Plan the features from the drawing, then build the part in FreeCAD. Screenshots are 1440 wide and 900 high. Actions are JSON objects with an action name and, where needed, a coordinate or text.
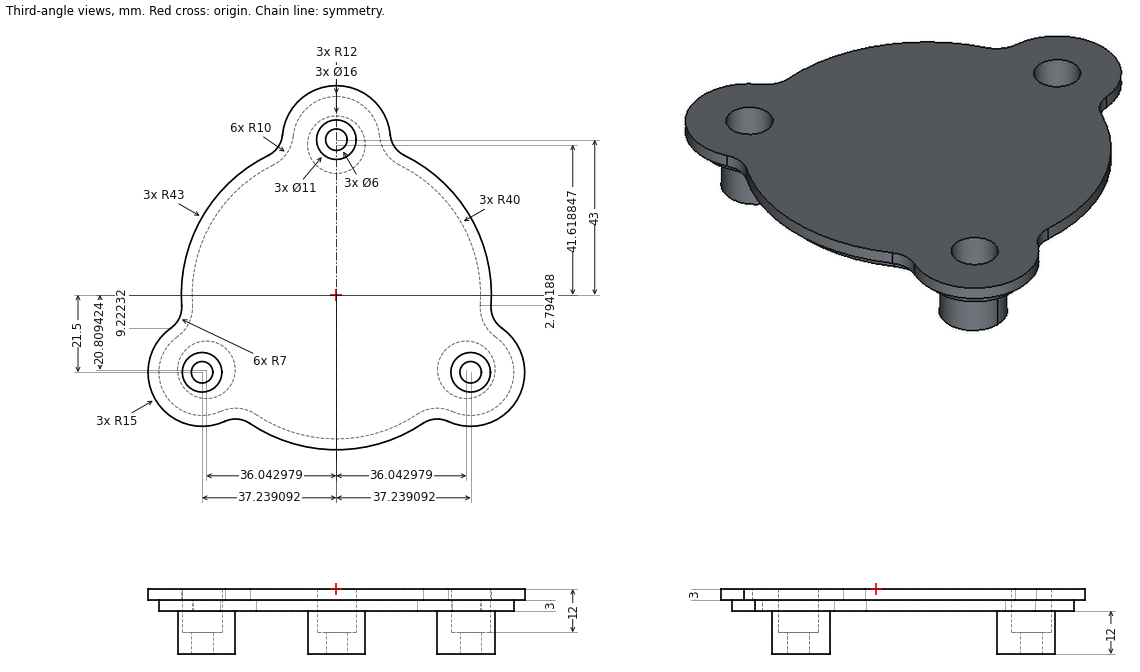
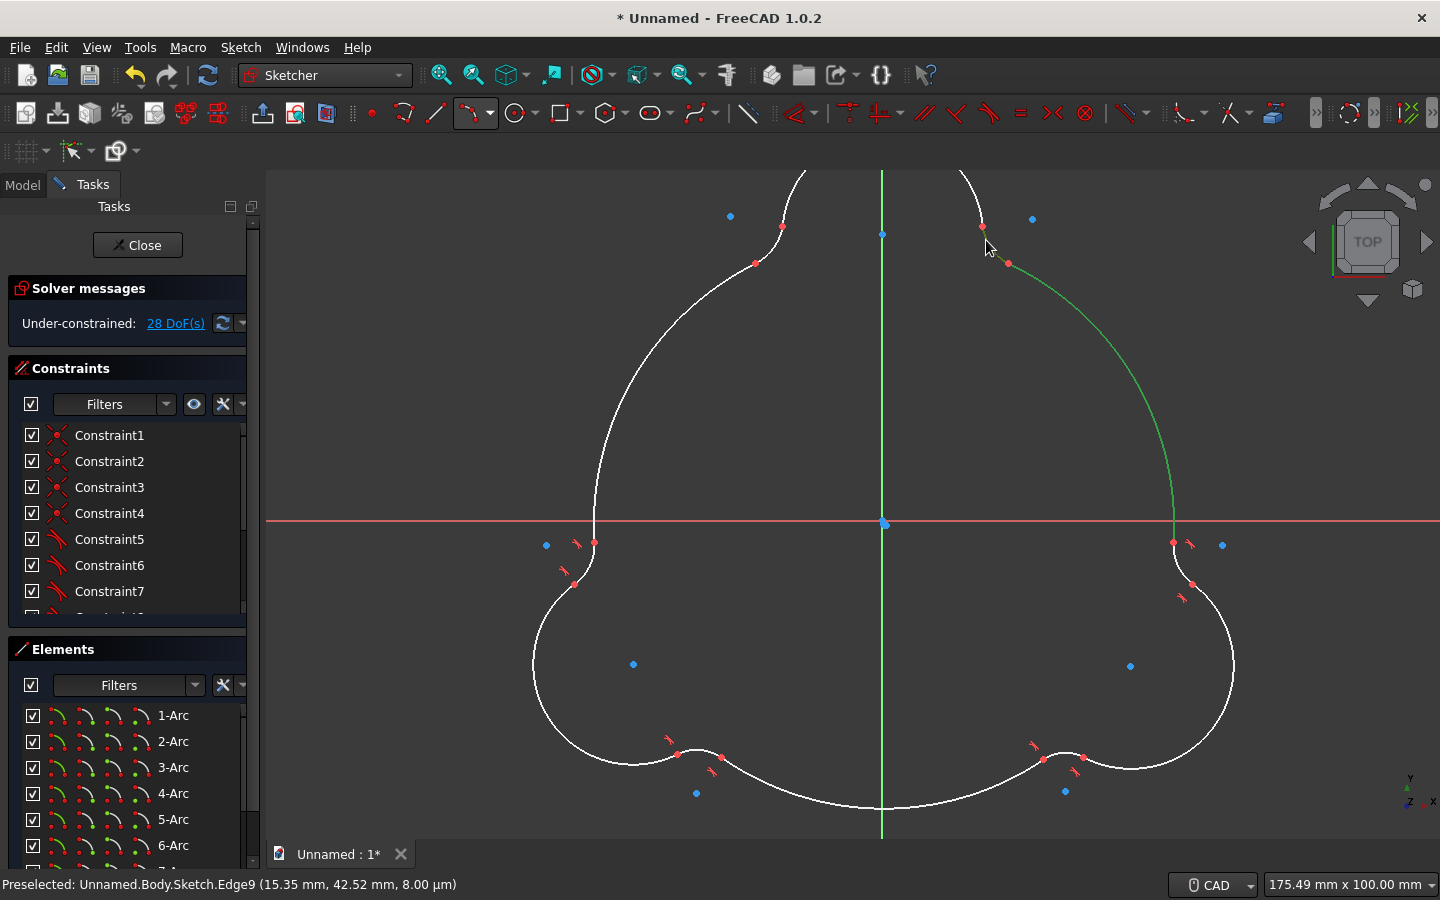
{"action": "left_click", "coordinate": [990, 114]}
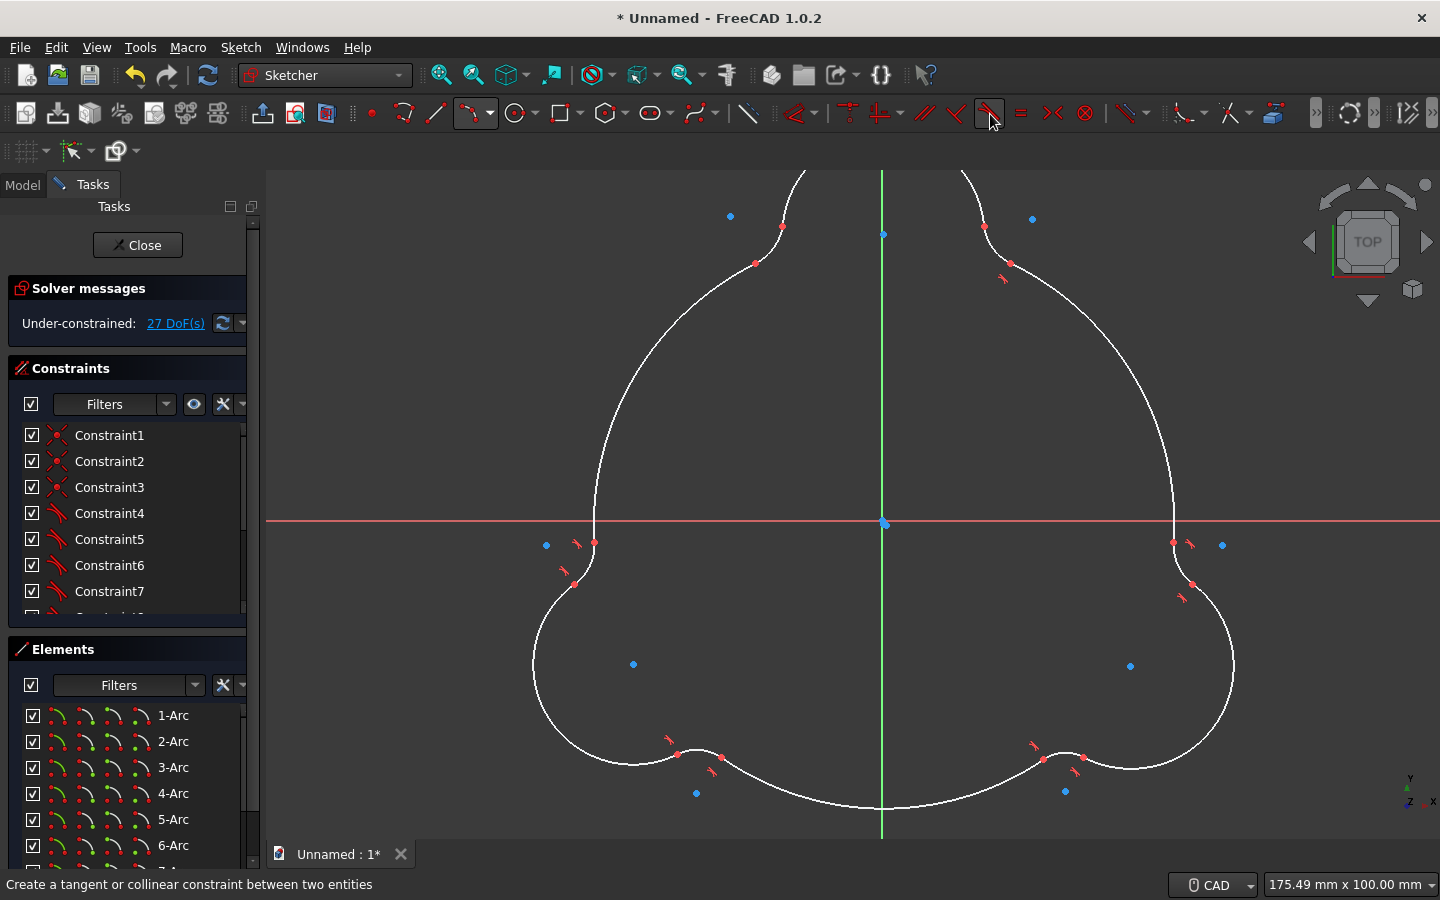
{"action": "left_click", "coordinate": [988, 240]}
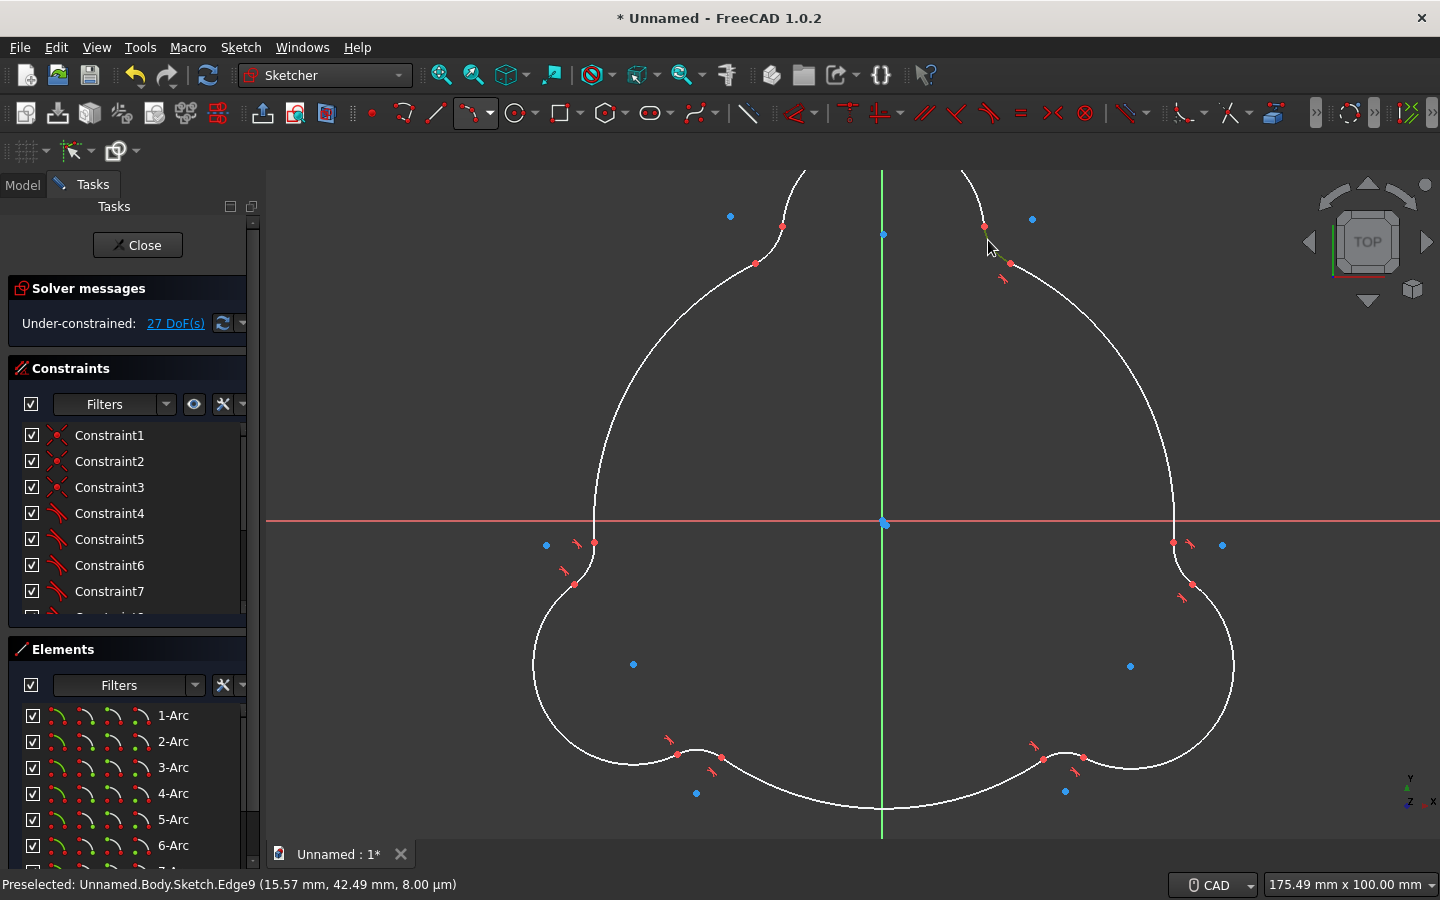
{"action": "scroll", "coordinate": [586, 574], "scroll_direction": "down", "scroll_amount": 2}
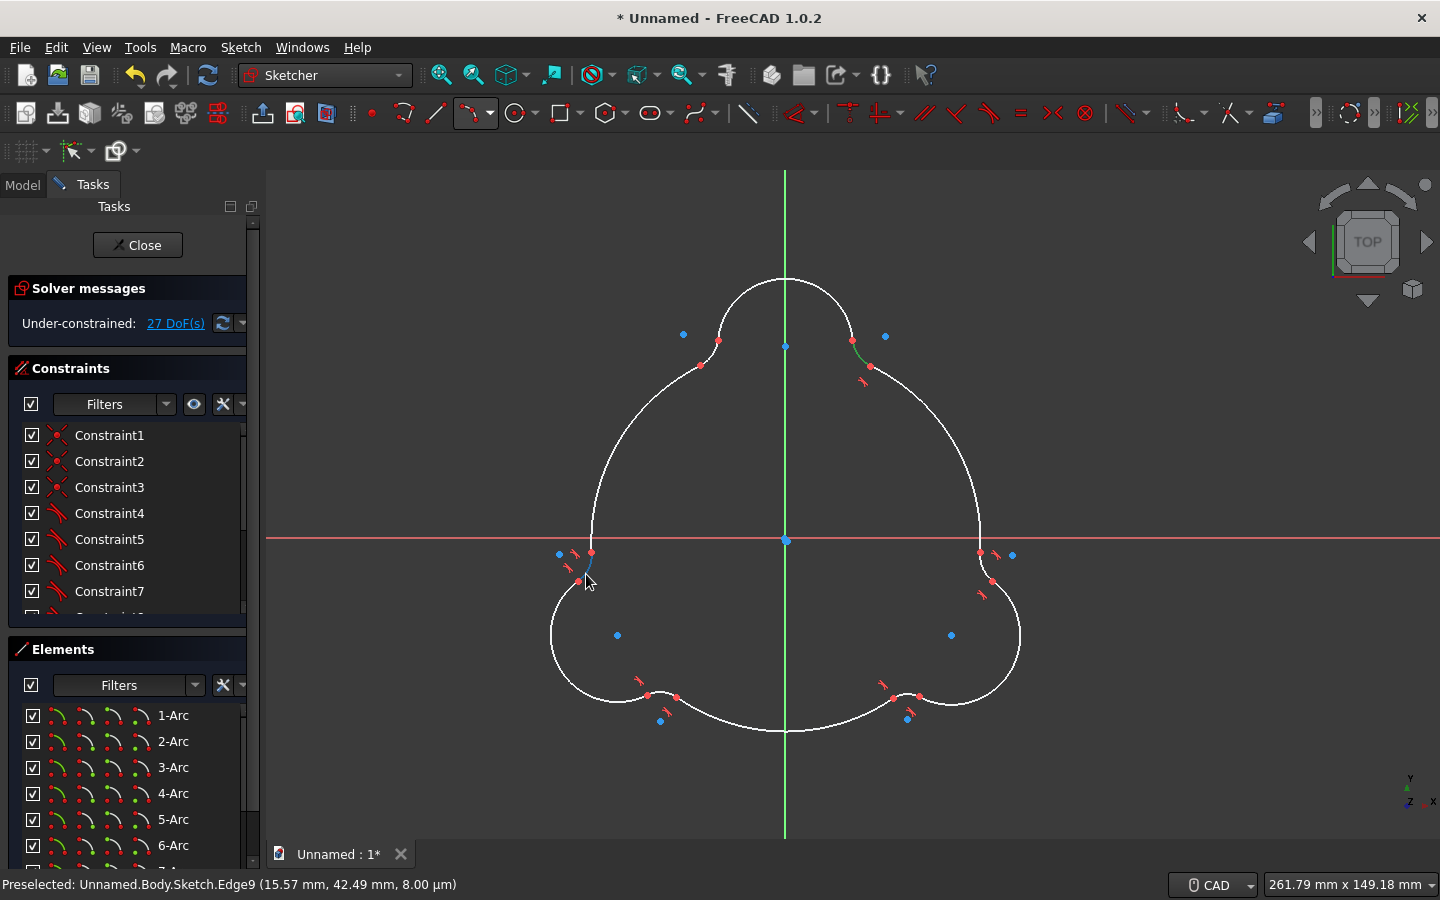
{"action": "left_click", "coordinate": [823, 290]}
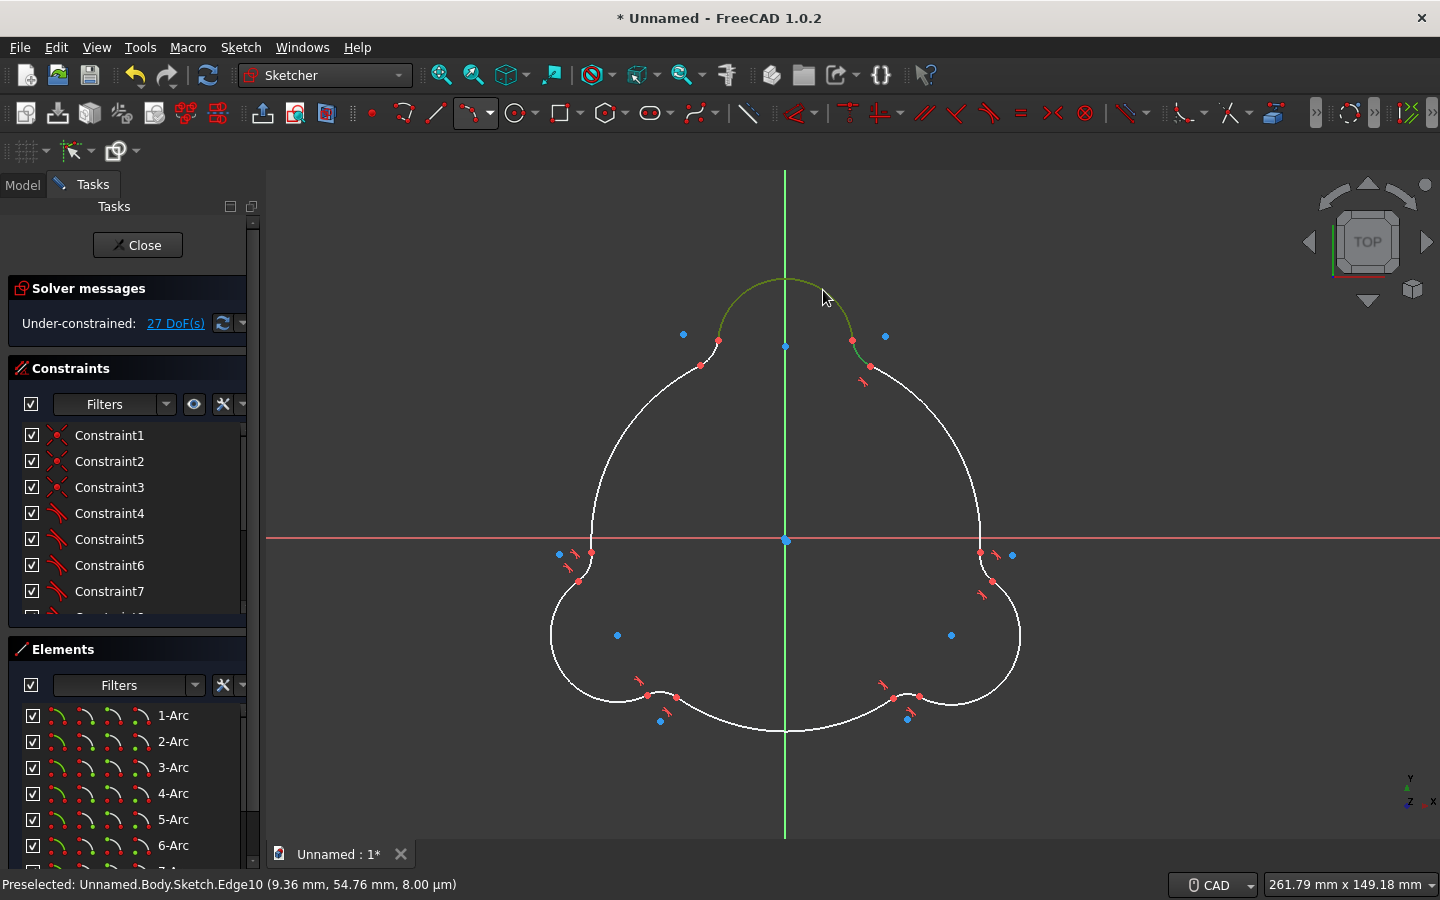
{"action": "left_click", "coordinate": [990, 114]}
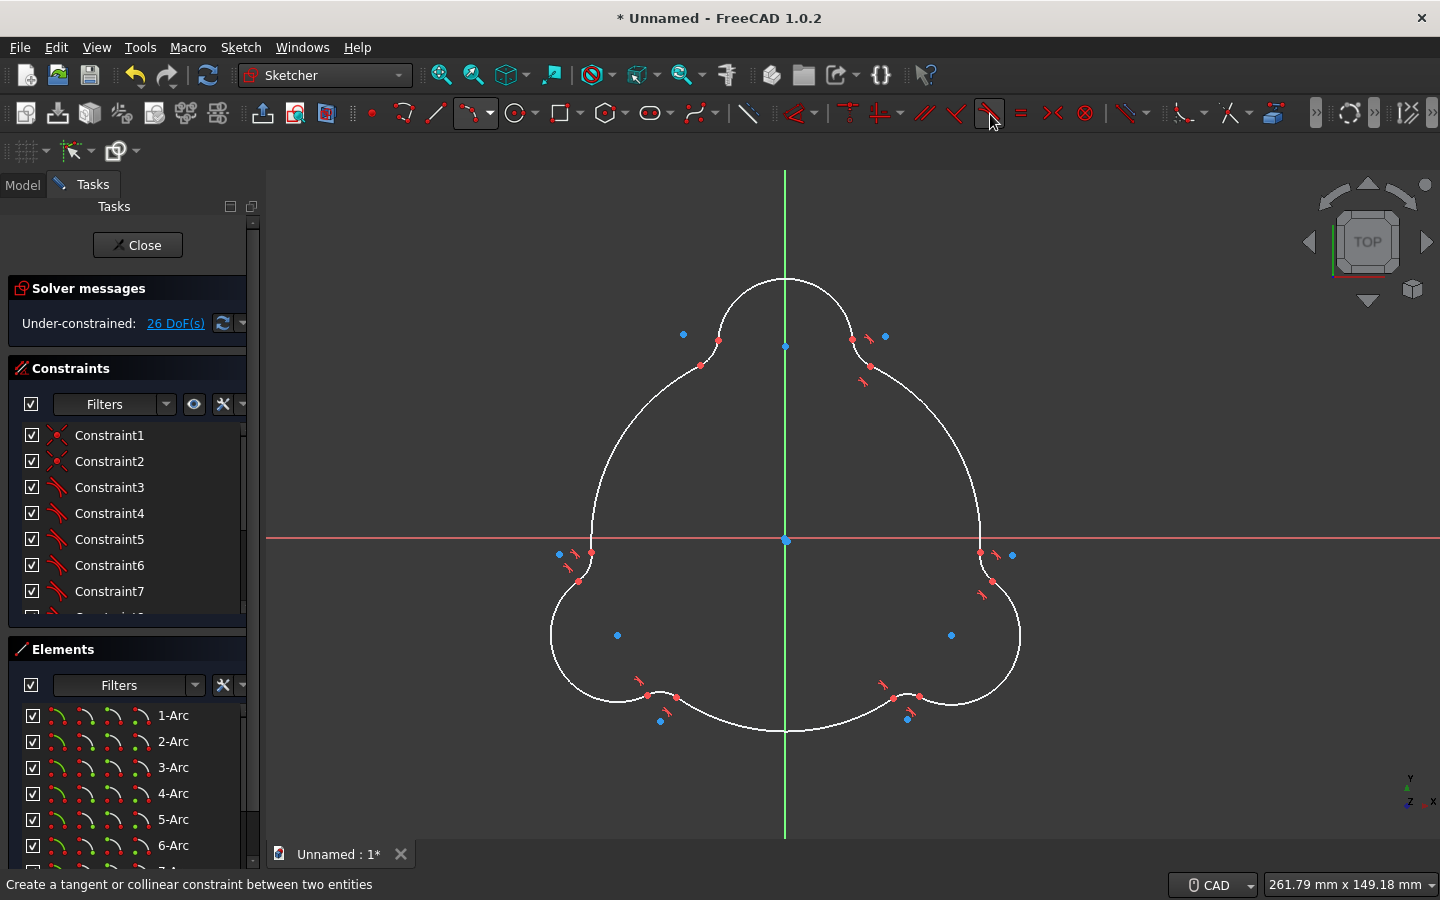
{"action": "left_click", "coordinate": [823, 290]}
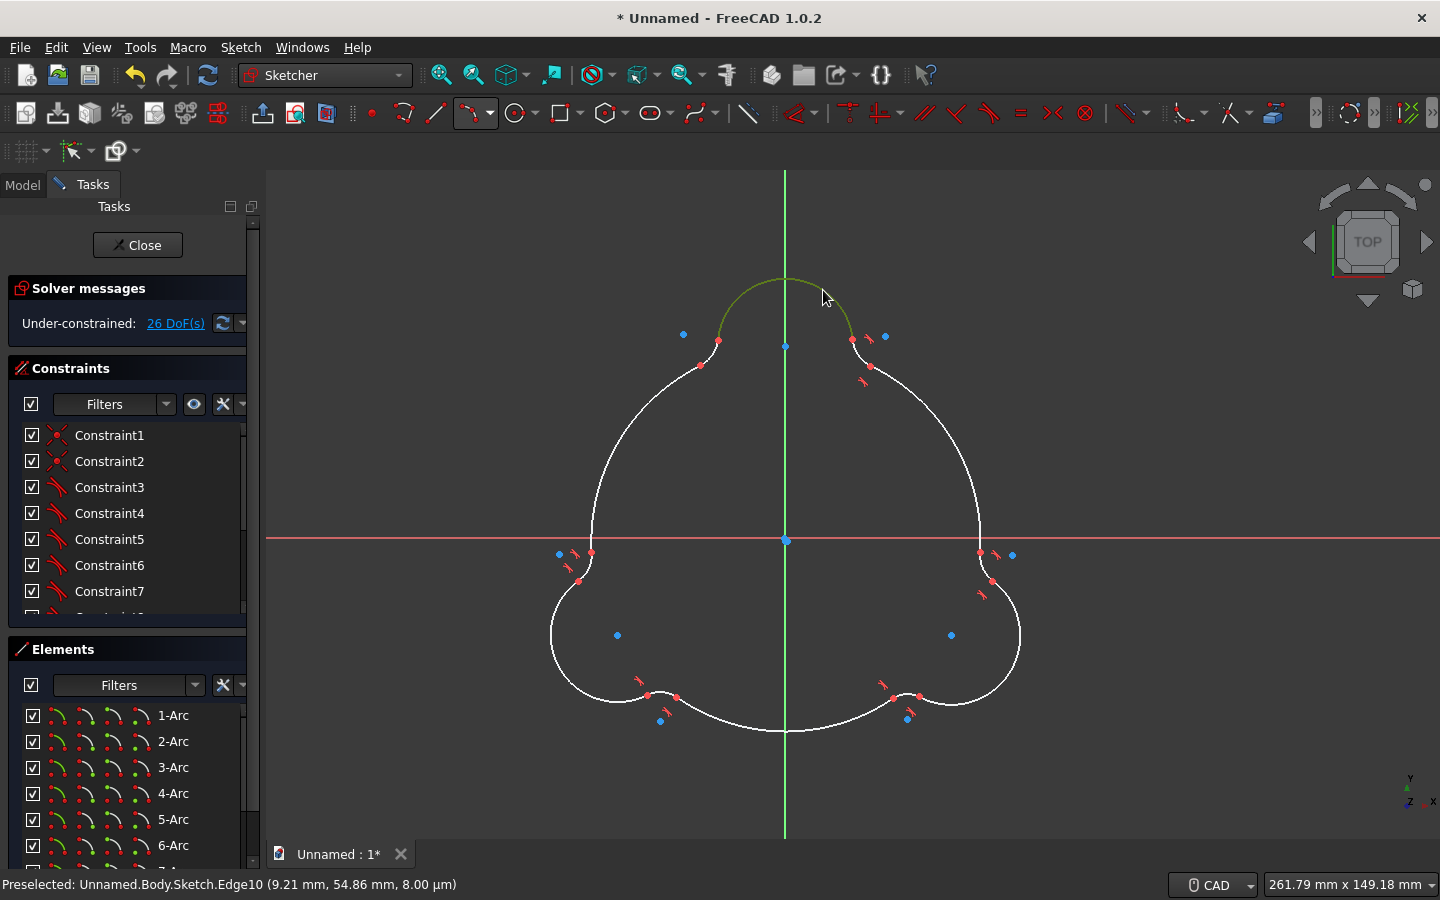
{"action": "scroll", "coordinate": [708, 360], "scroll_direction": "up", "scroll_amount": 2}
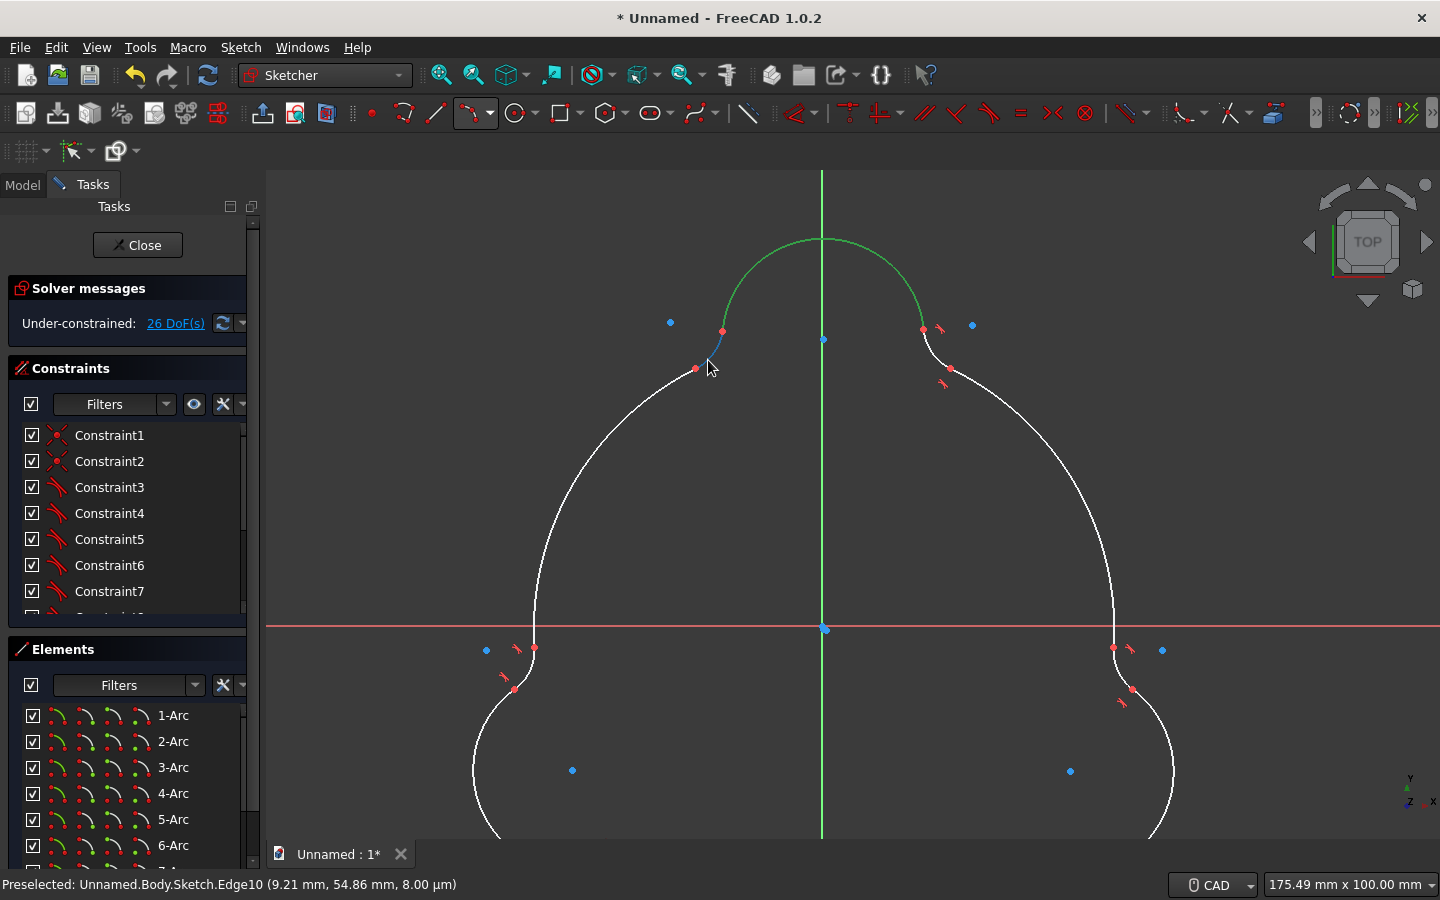
{"action": "left_click", "coordinate": [707, 360]}